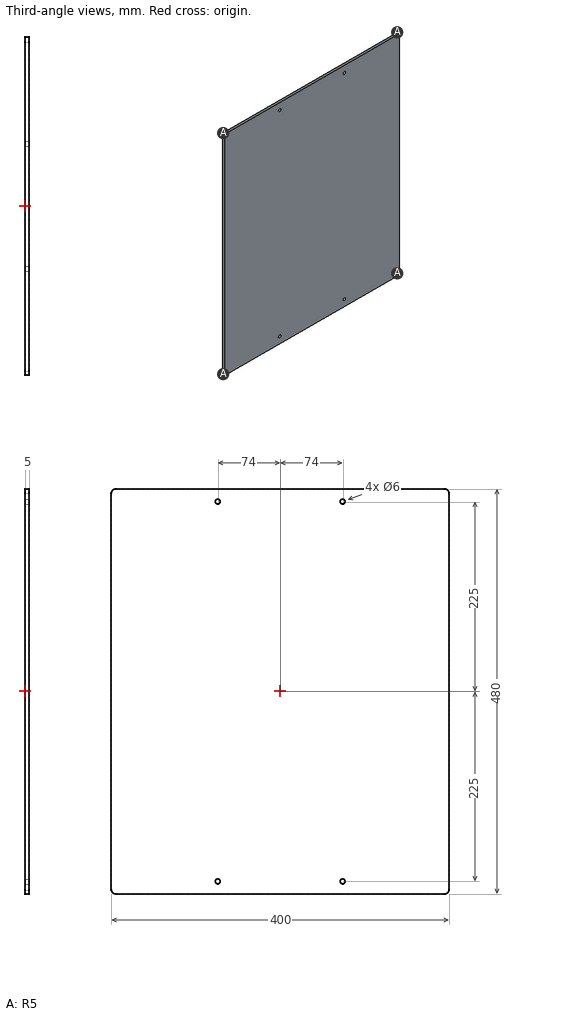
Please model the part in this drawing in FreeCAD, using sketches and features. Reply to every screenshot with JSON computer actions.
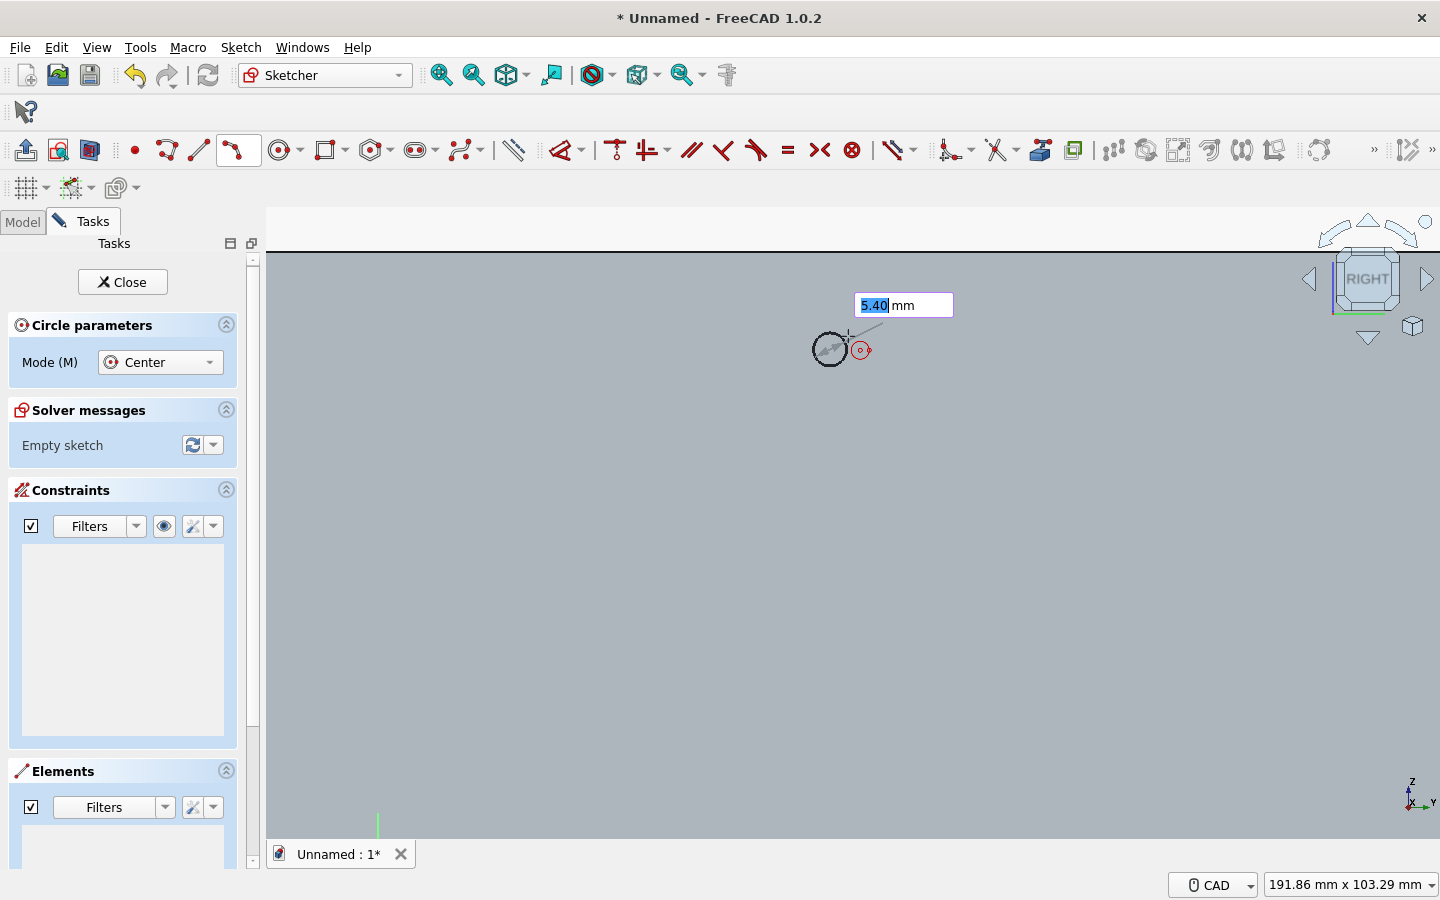
{"action": "left_click", "coordinate": [844, 331]}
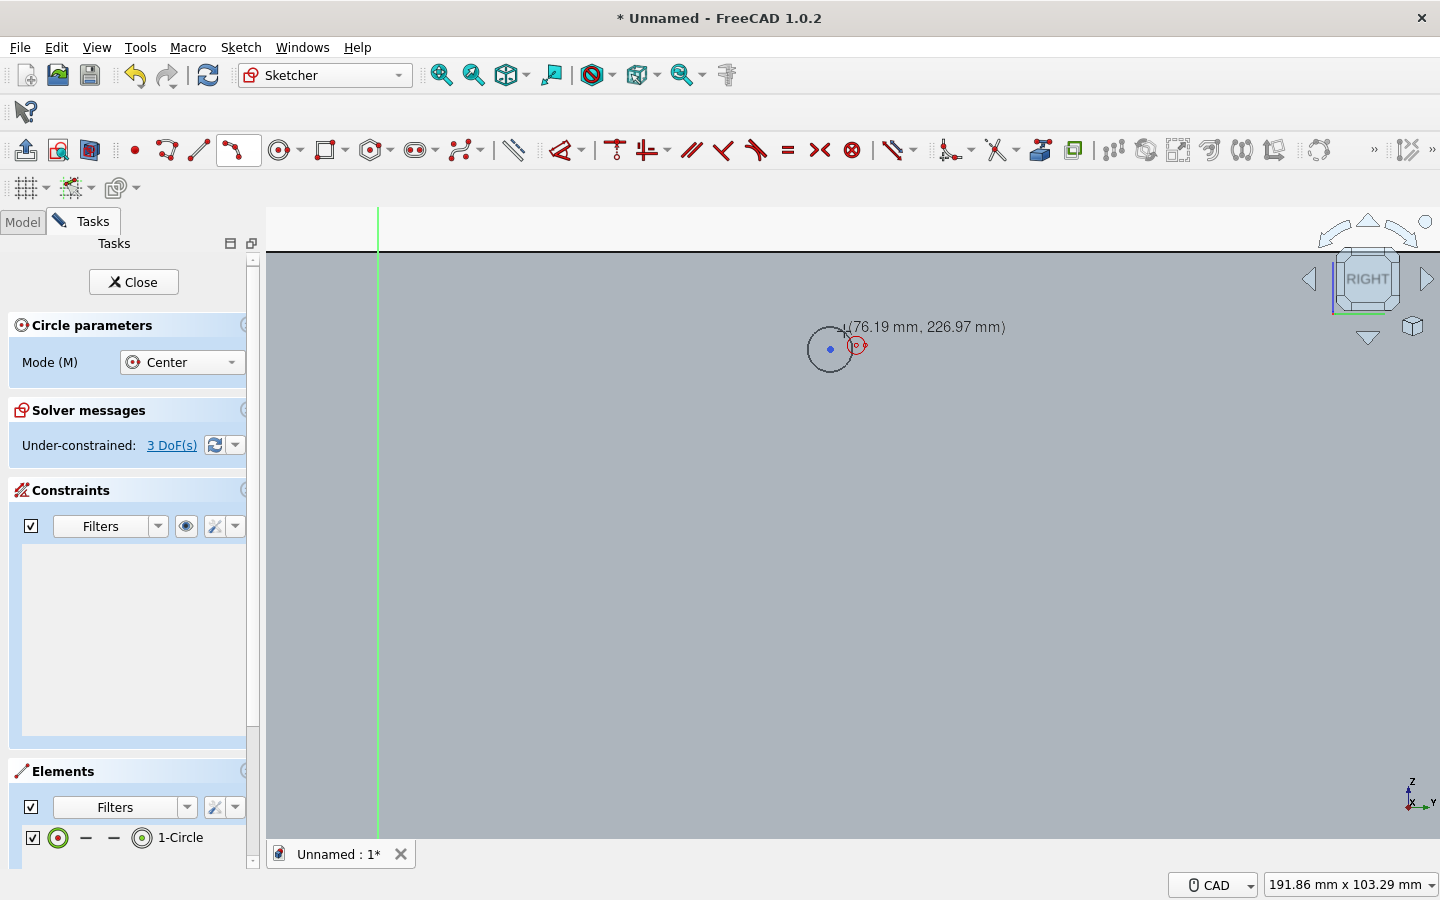
{"action": "scroll", "coordinate": [848, 336], "scroll_direction": "down", "scroll_amount": 10}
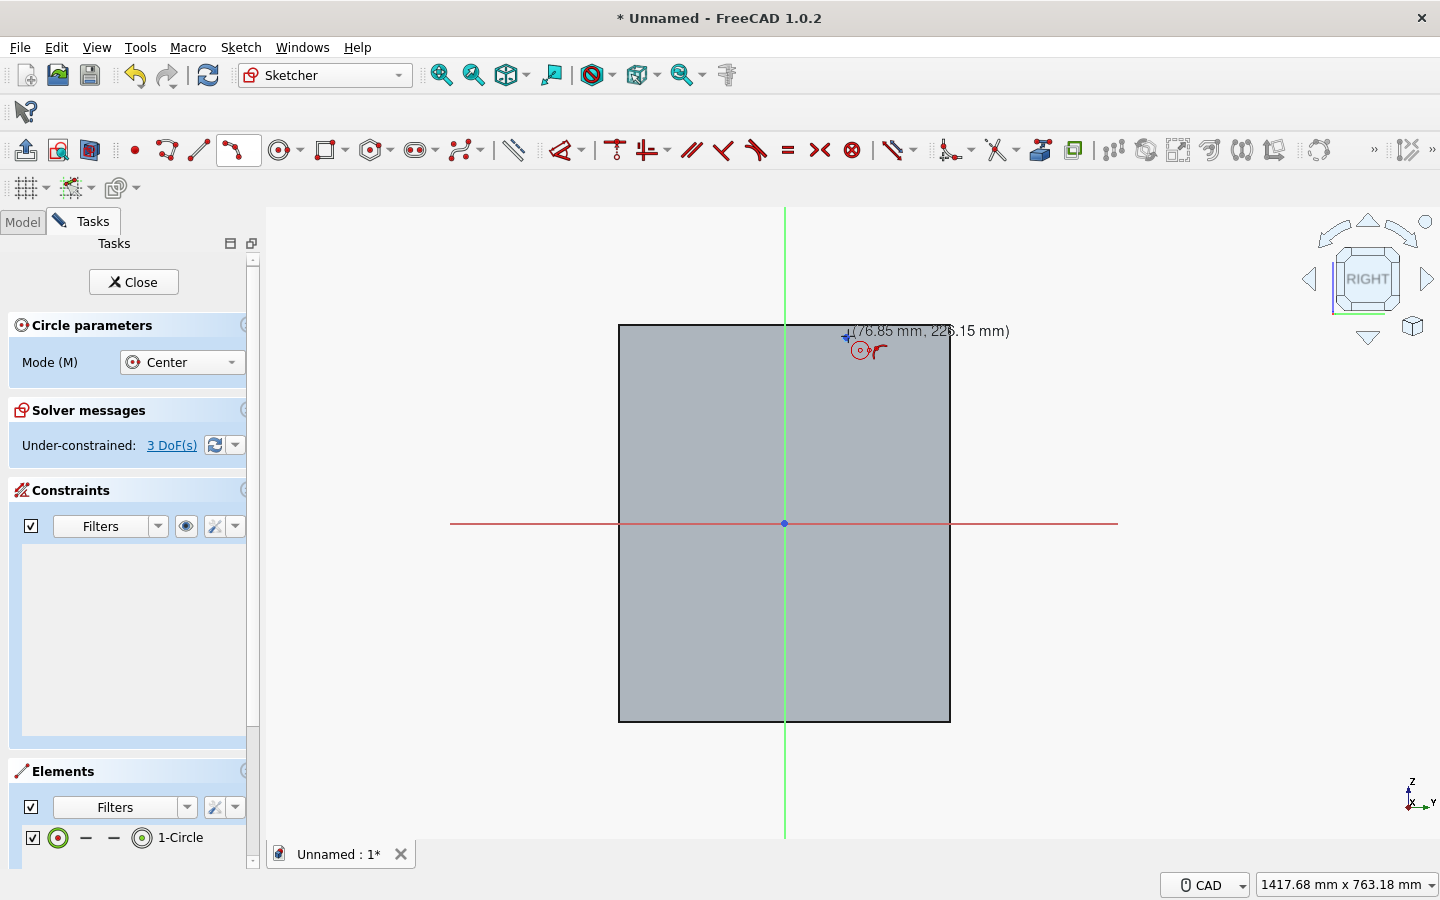
{"action": "scroll", "coordinate": [846, 710], "scroll_direction": "up", "scroll_amount": 12}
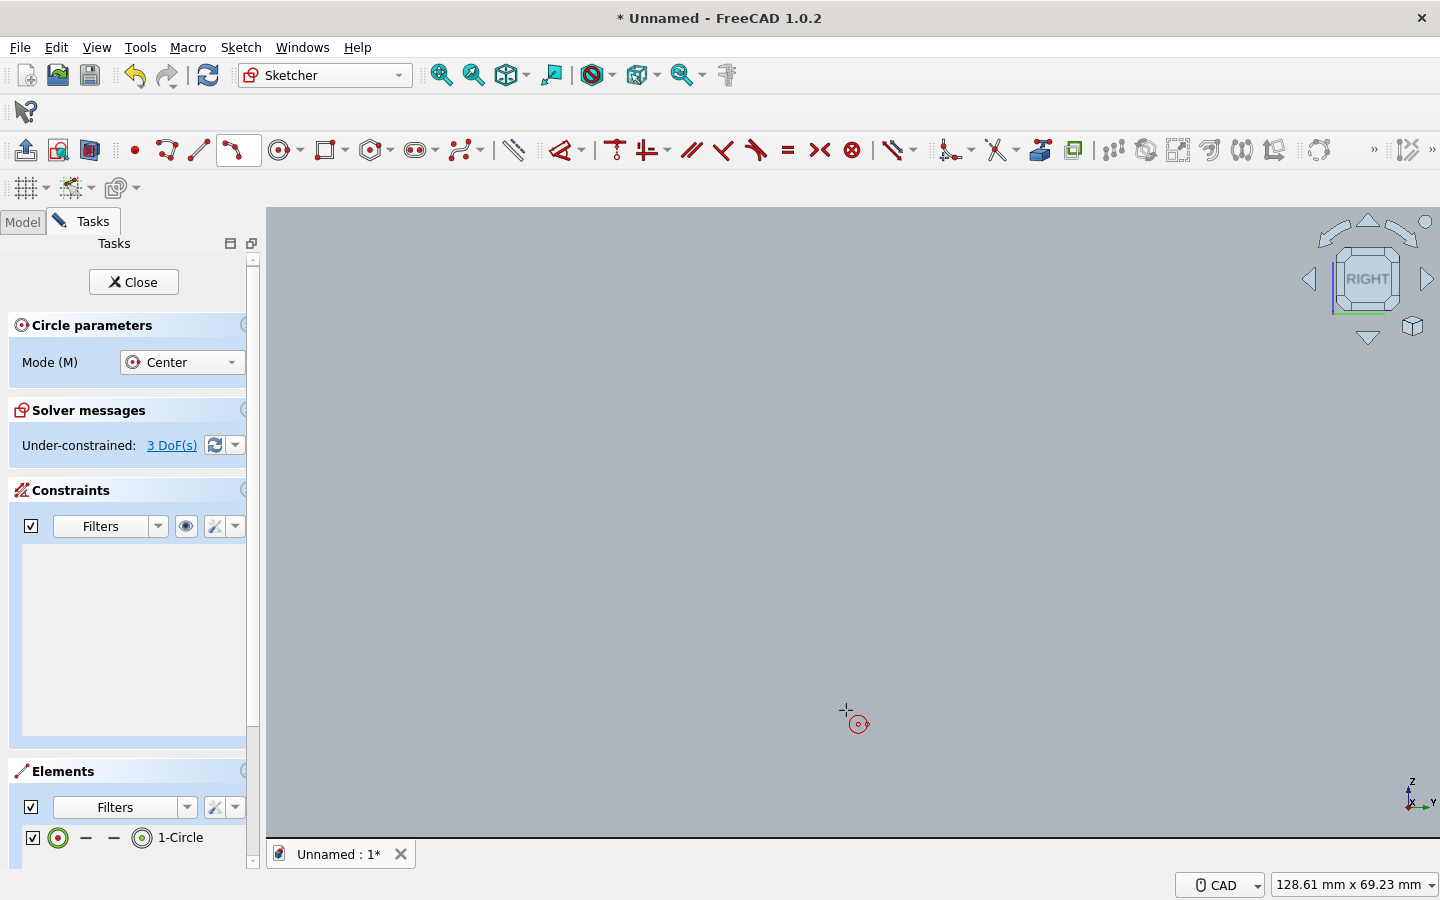
{"action": "scroll", "coordinate": [846, 710], "scroll_direction": "down", "scroll_amount": 12}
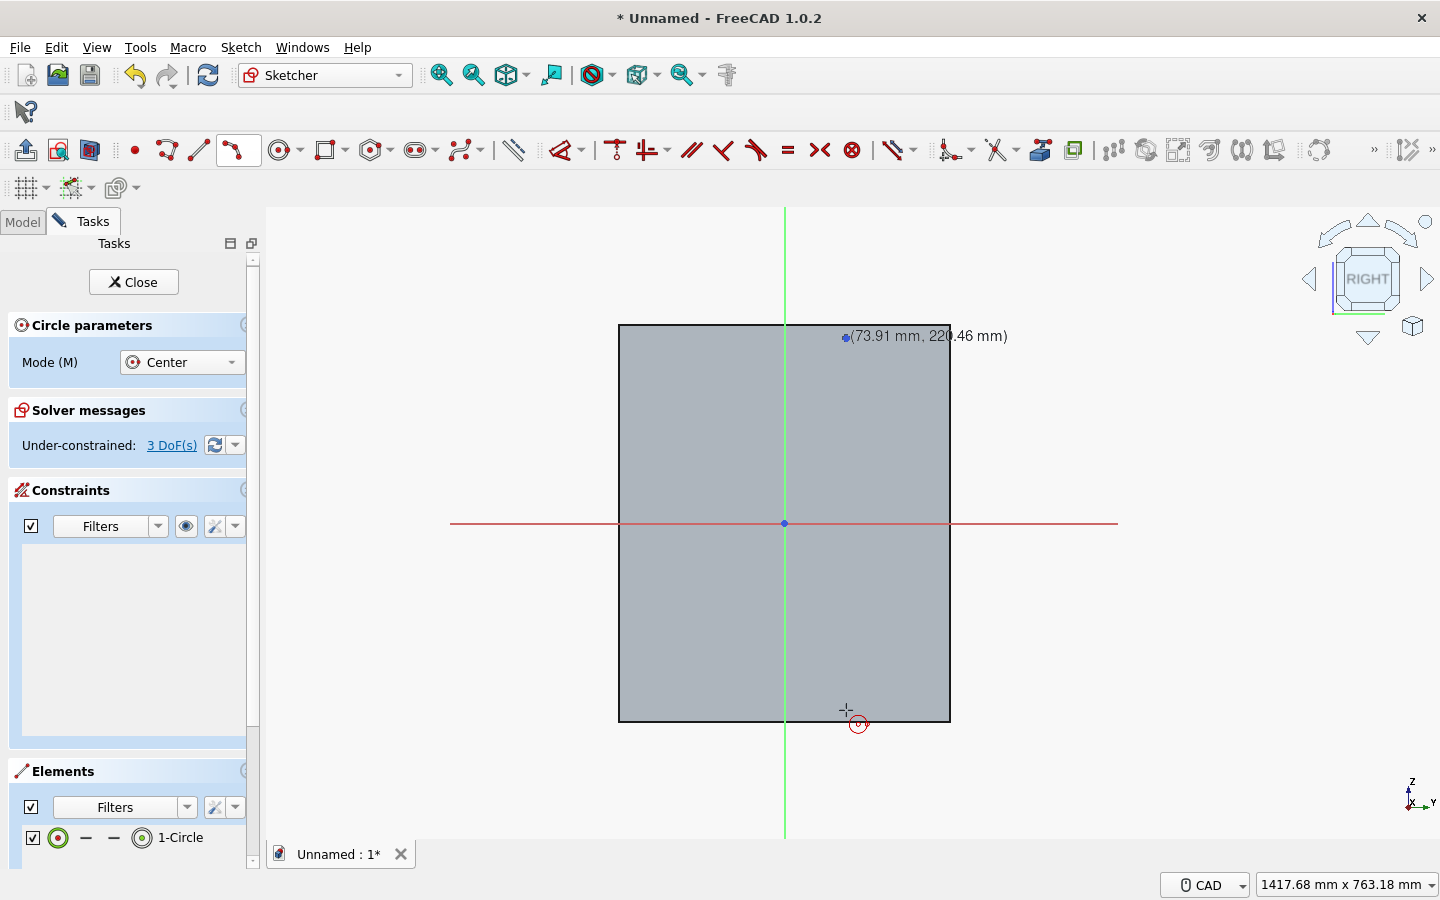
{"action": "left_click", "coordinate": [846, 710]}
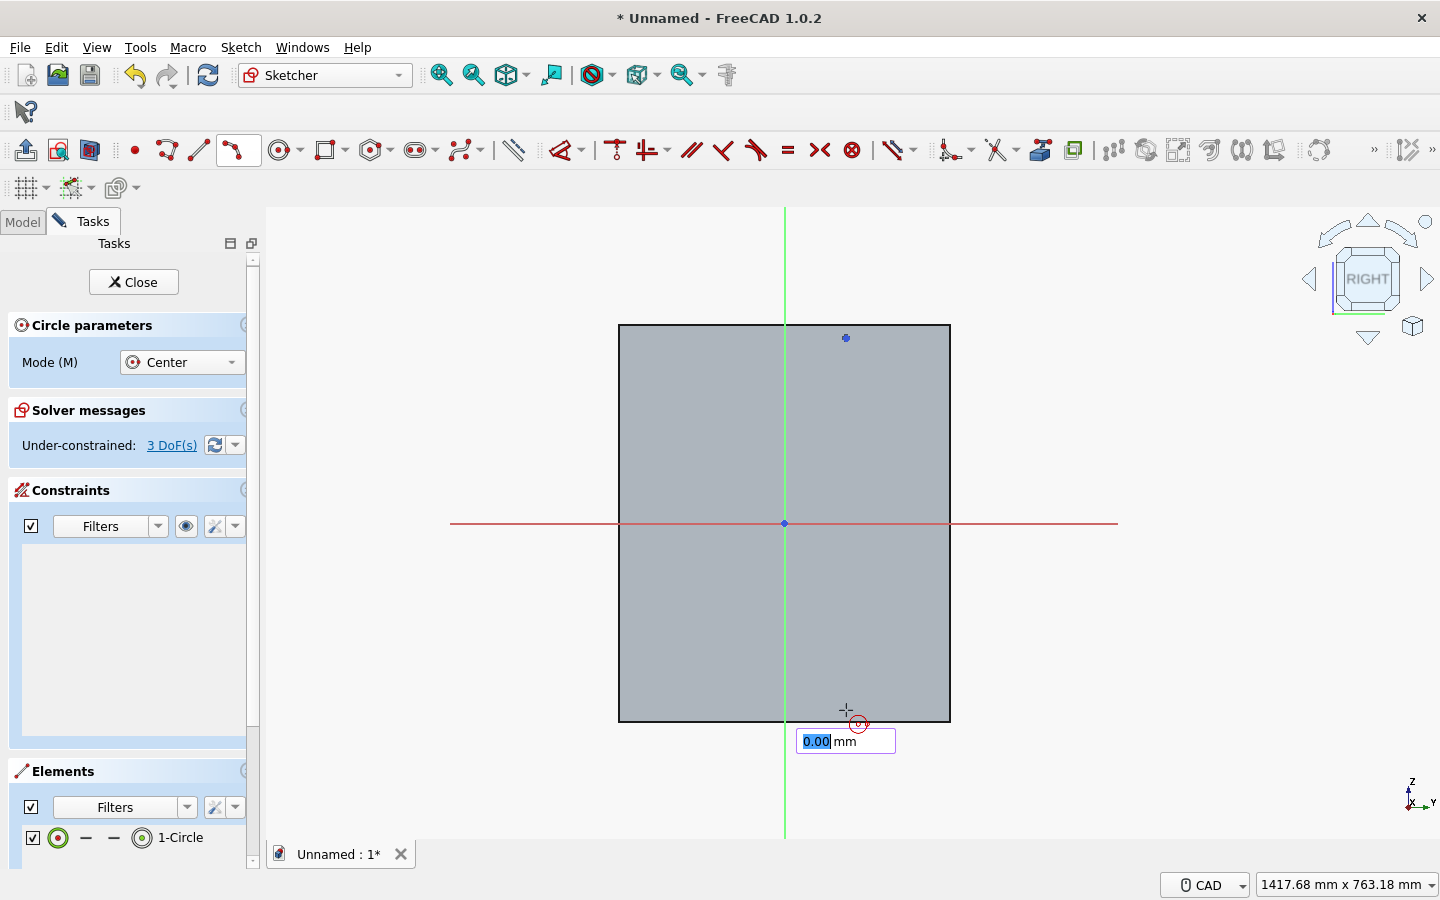
{"action": "scroll", "coordinate": [848, 708], "scroll_direction": "up", "scroll_amount": 10}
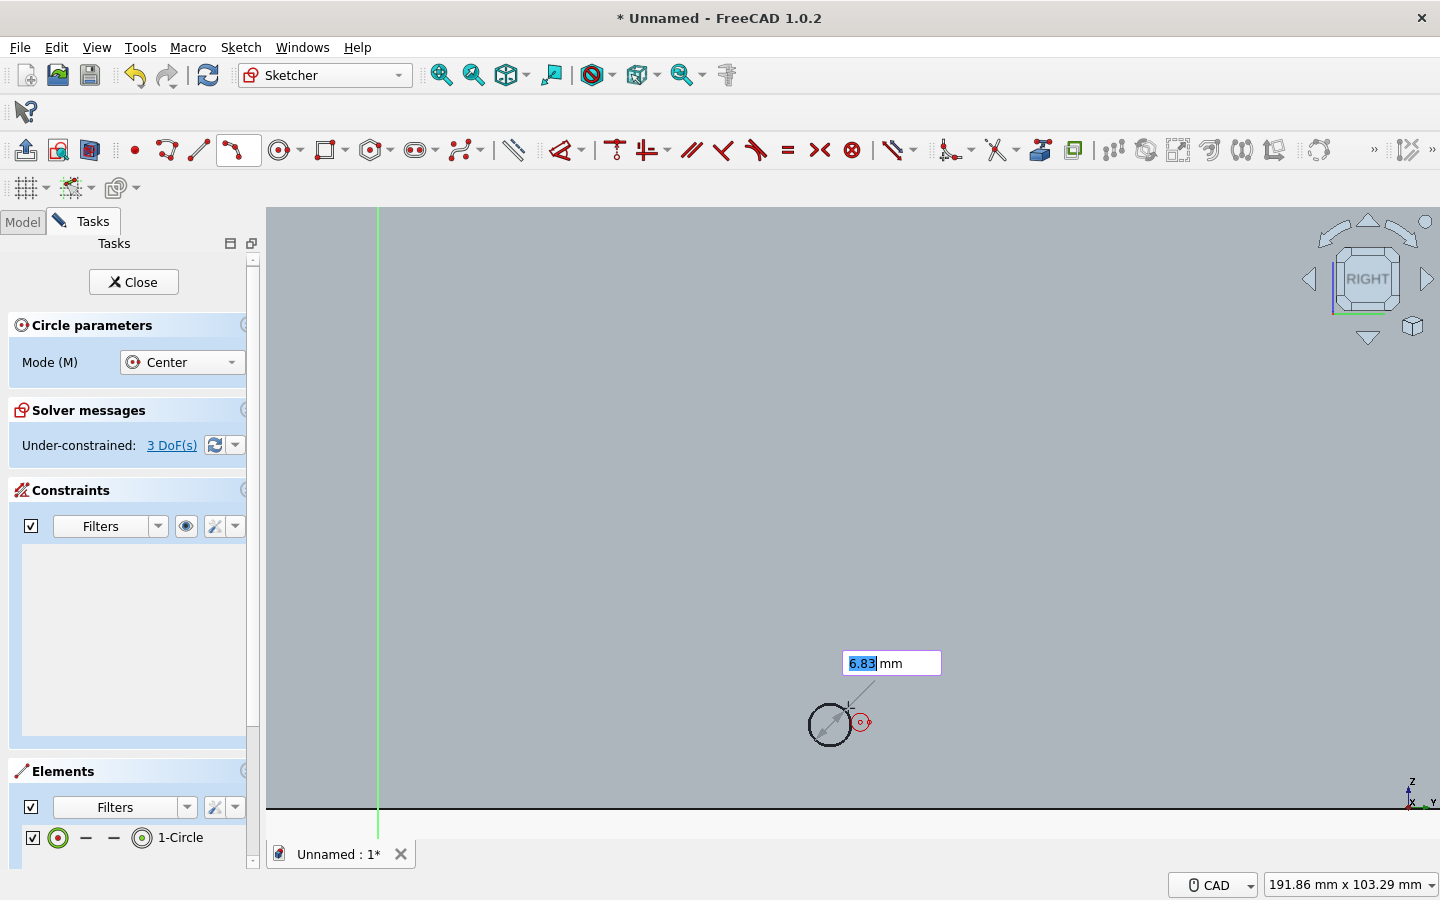
{"action": "left_click", "coordinate": [844, 704]}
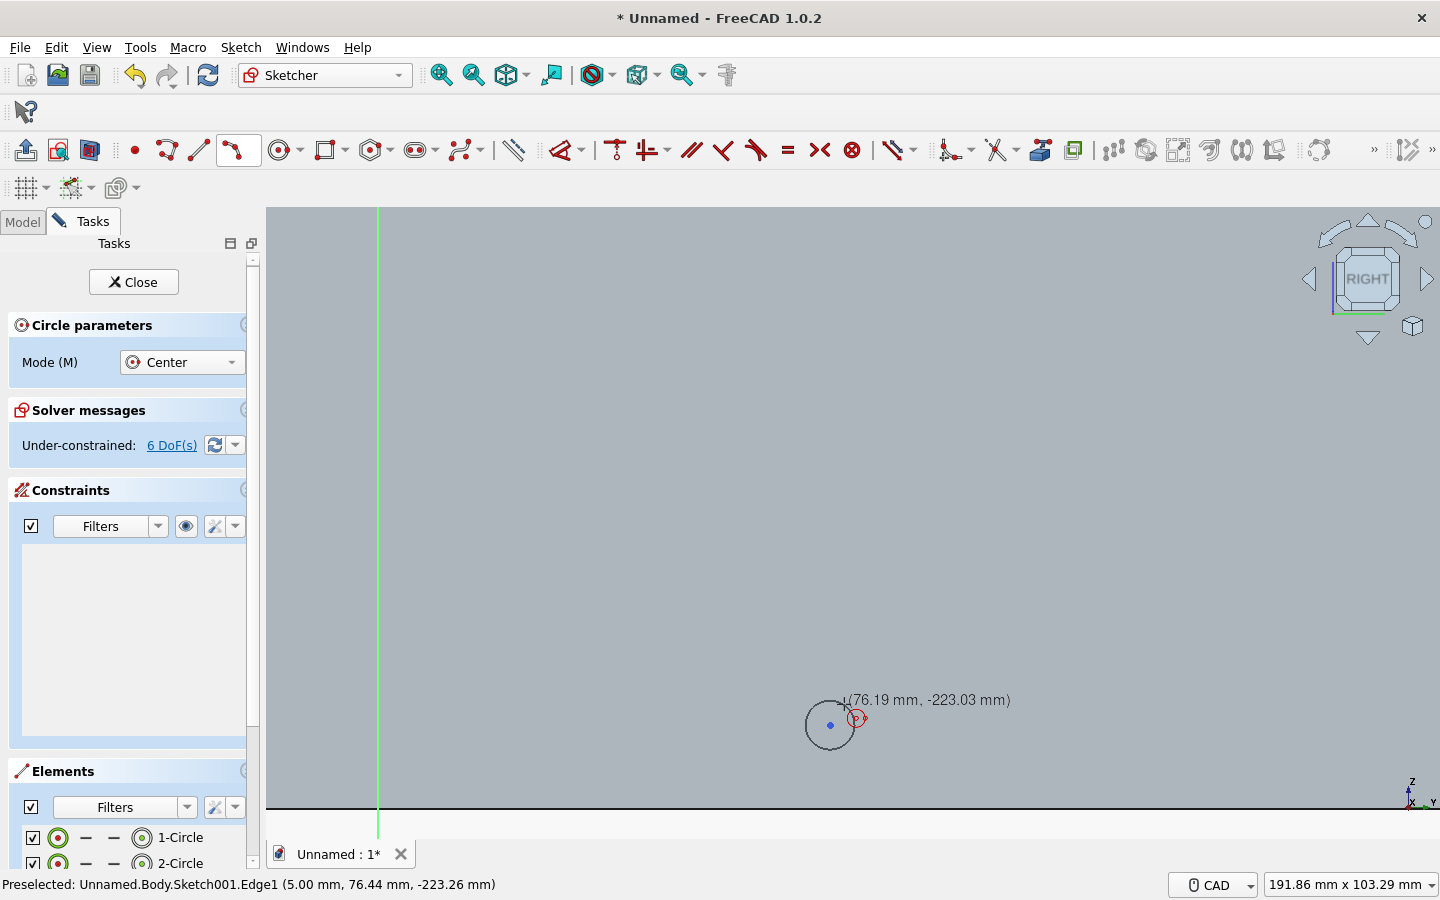
{"action": "scroll", "coordinate": [848, 708], "scroll_direction": "down", "scroll_amount": 10}